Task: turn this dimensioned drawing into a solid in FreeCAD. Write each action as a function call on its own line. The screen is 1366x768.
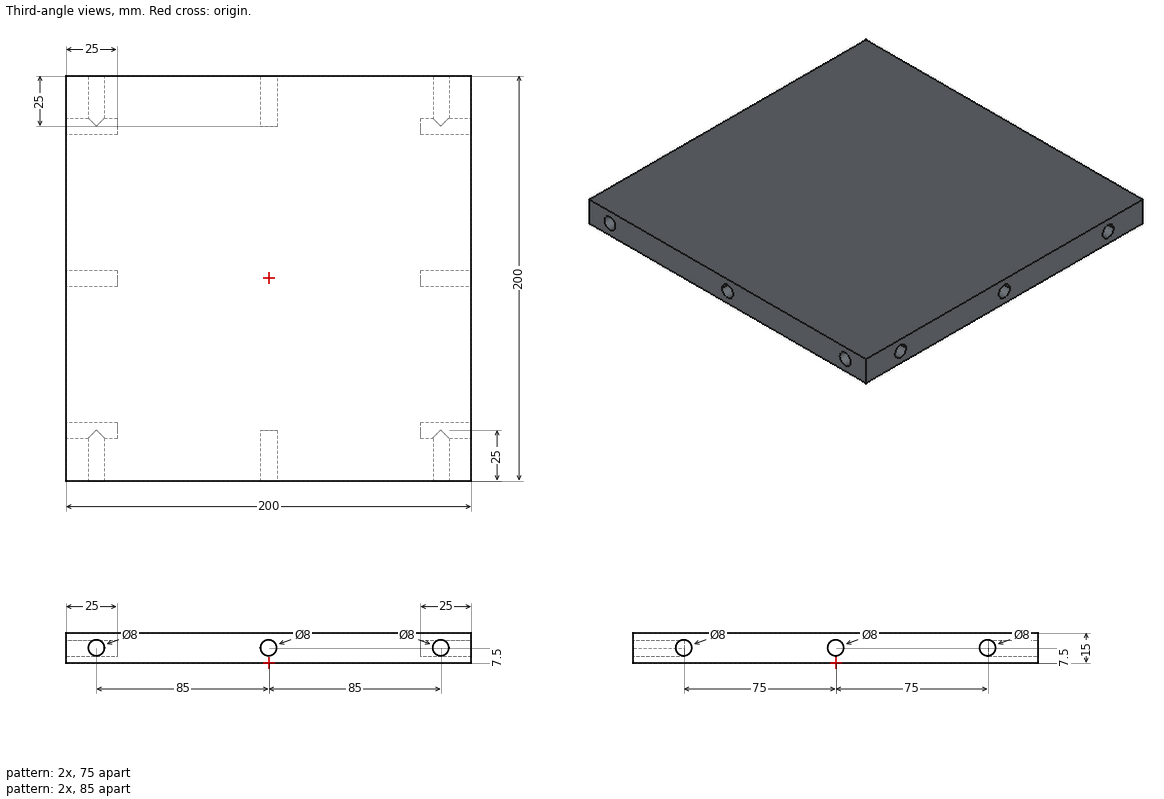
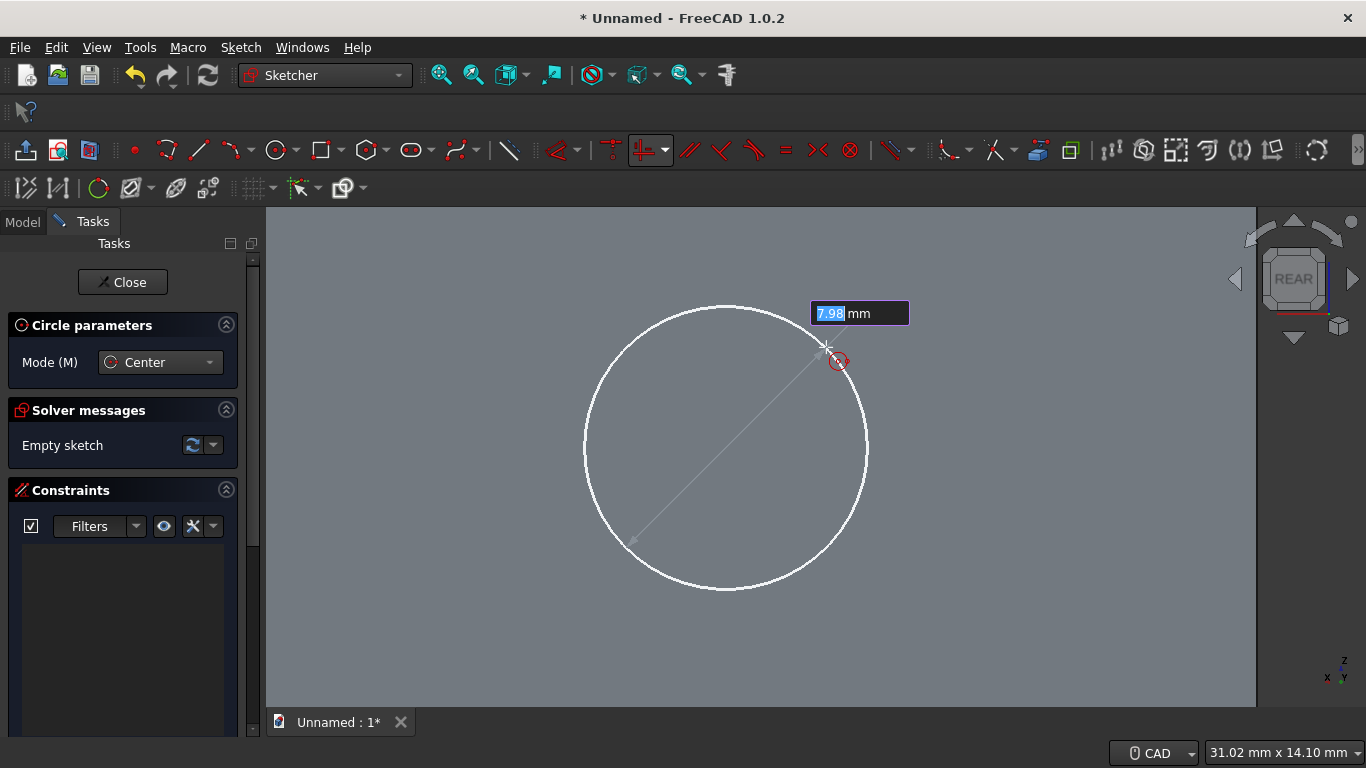
text(8)
key(Return)
key(Escape)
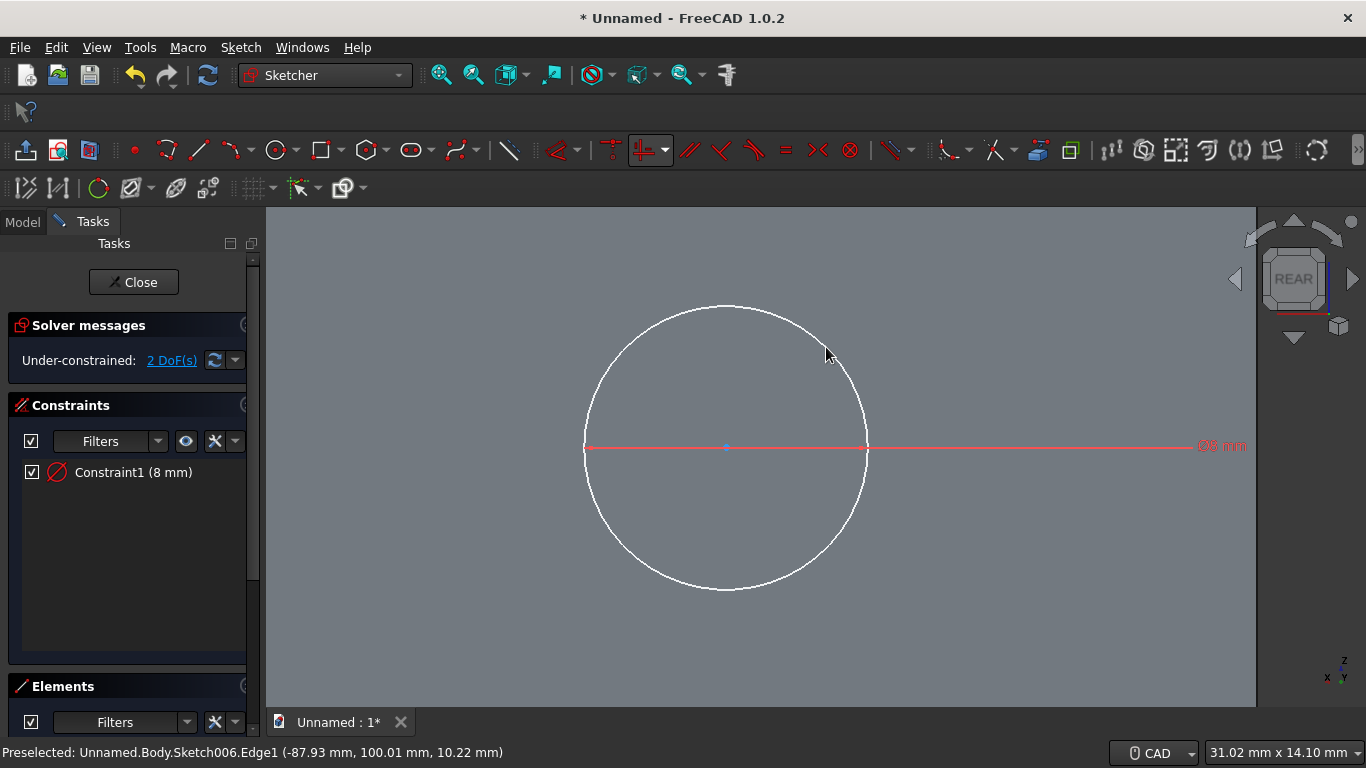
key(d)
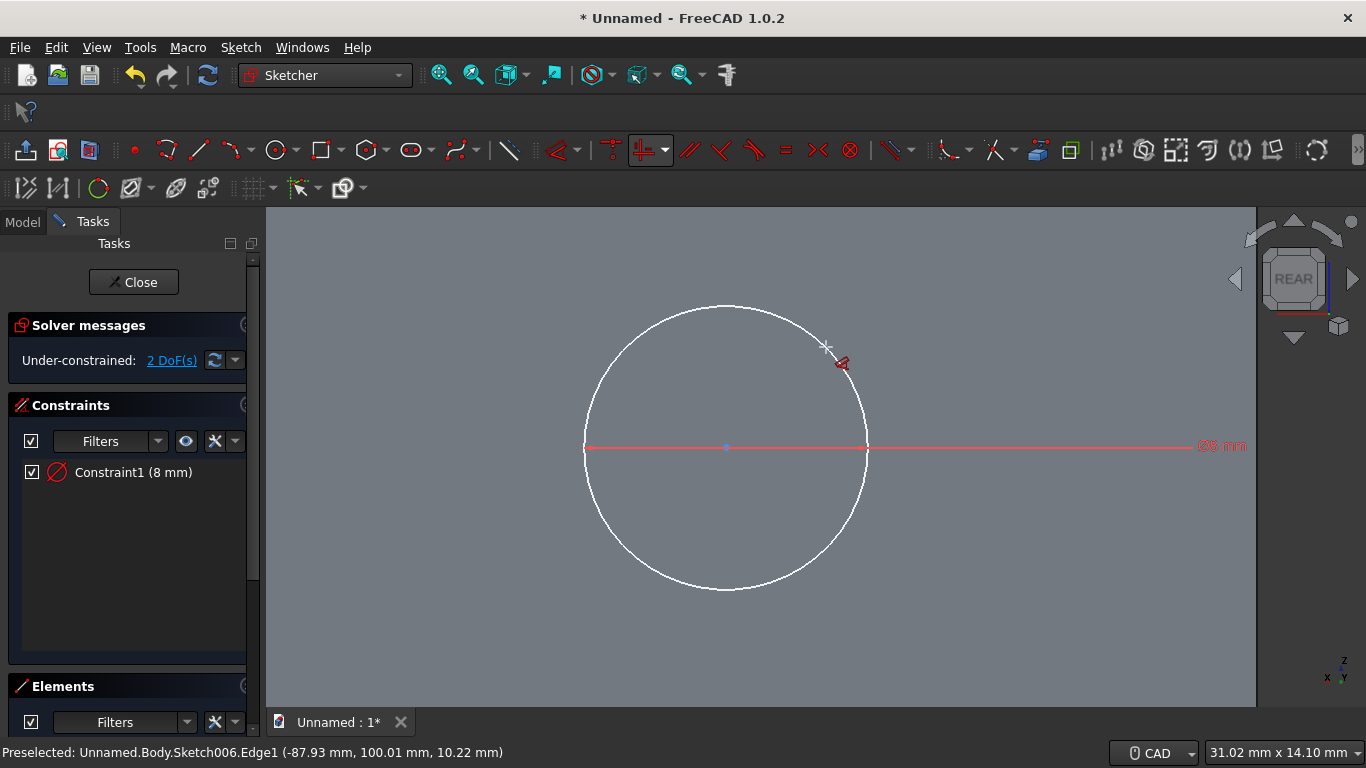
click(726, 448)
click(510, 414)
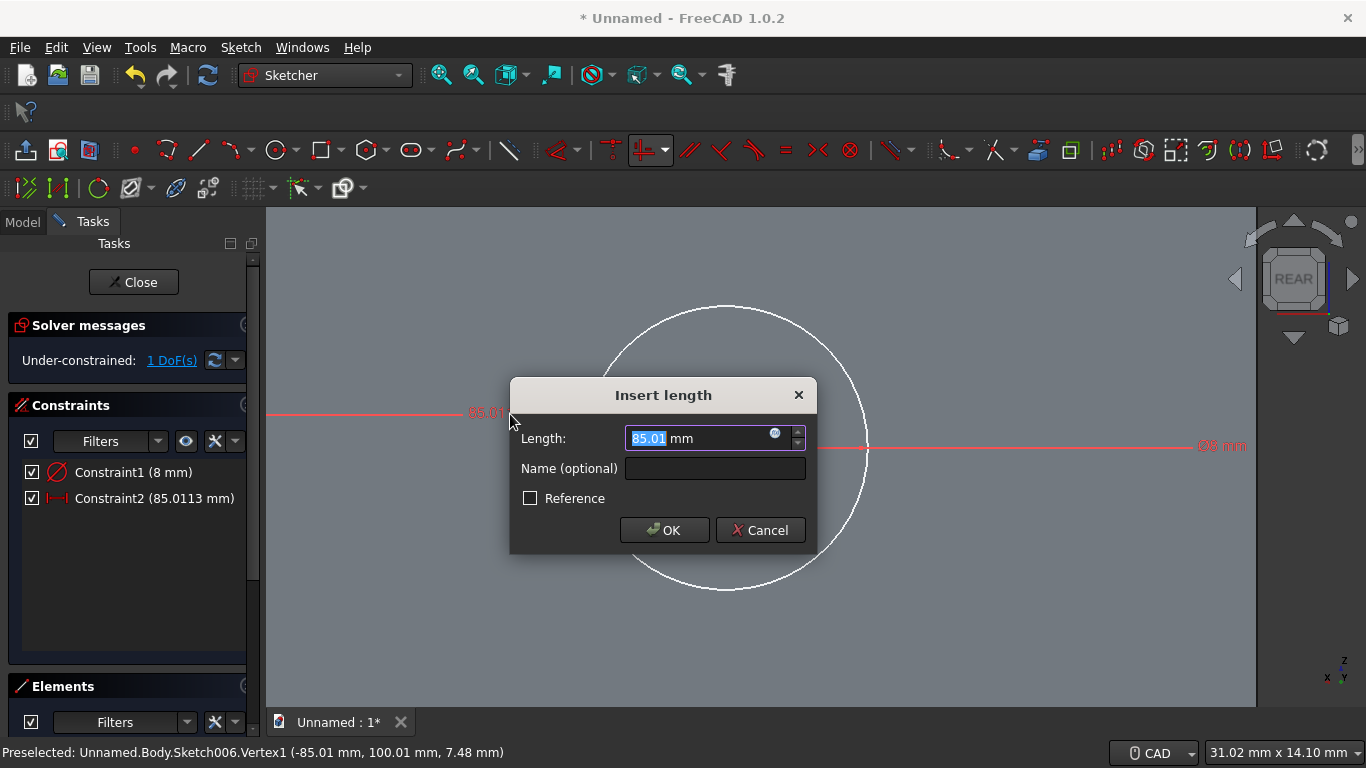
text(85)
key(Return)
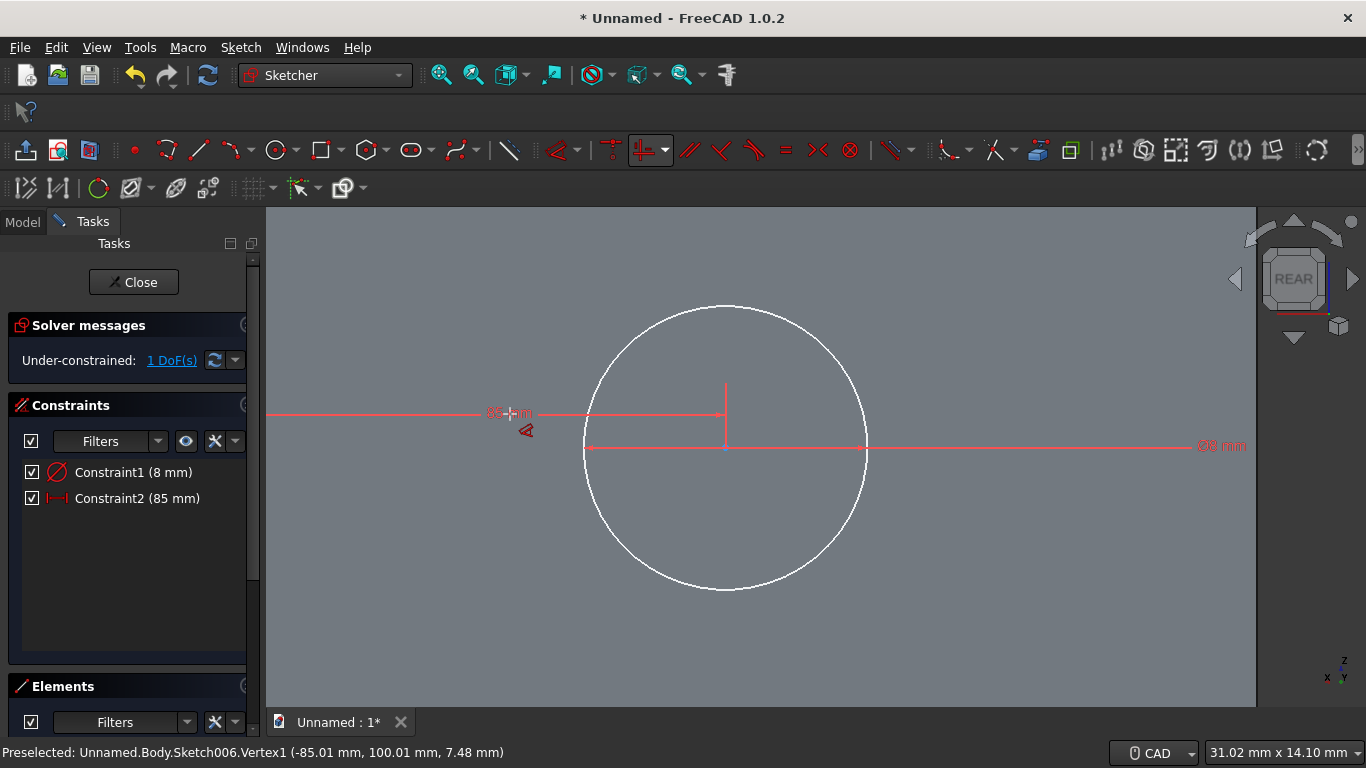
click(726, 448)
click(760, 563)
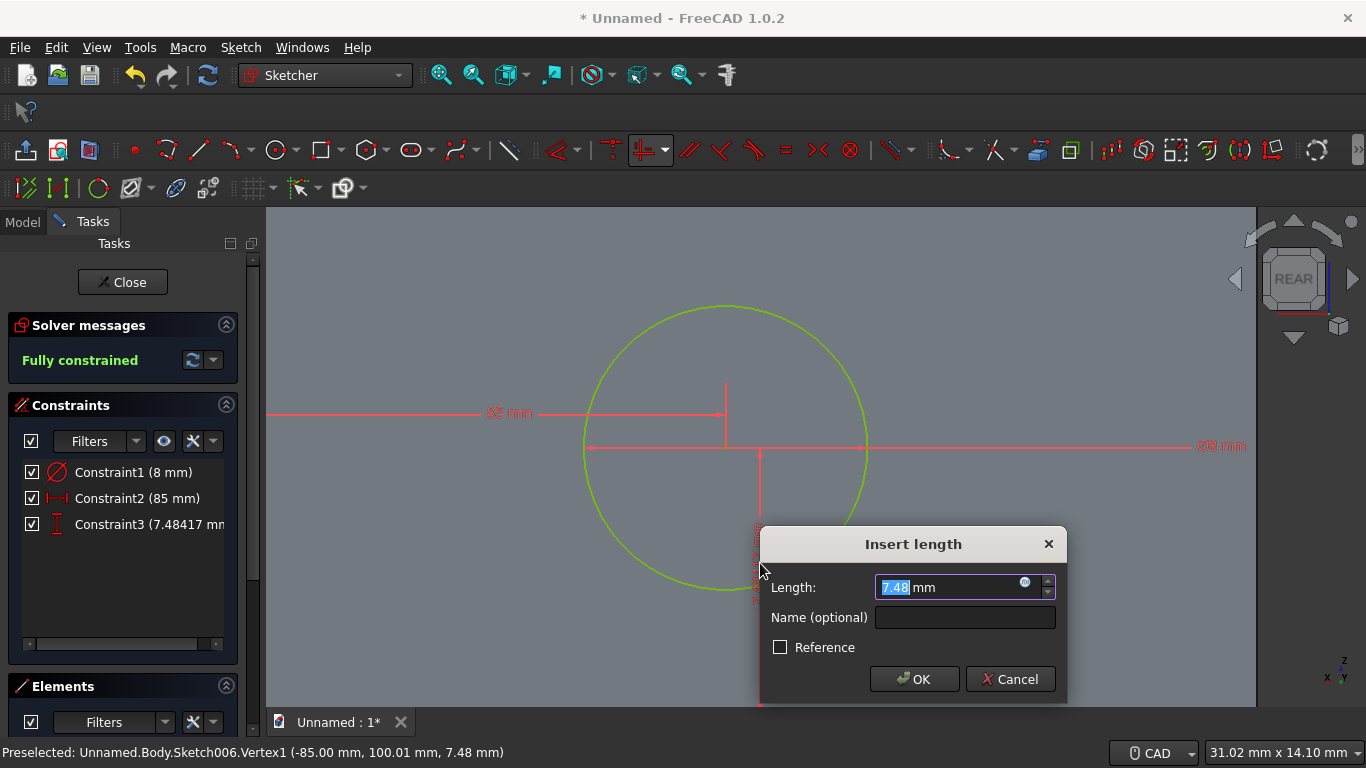
text(7.5)
key(Return)
key(Escape)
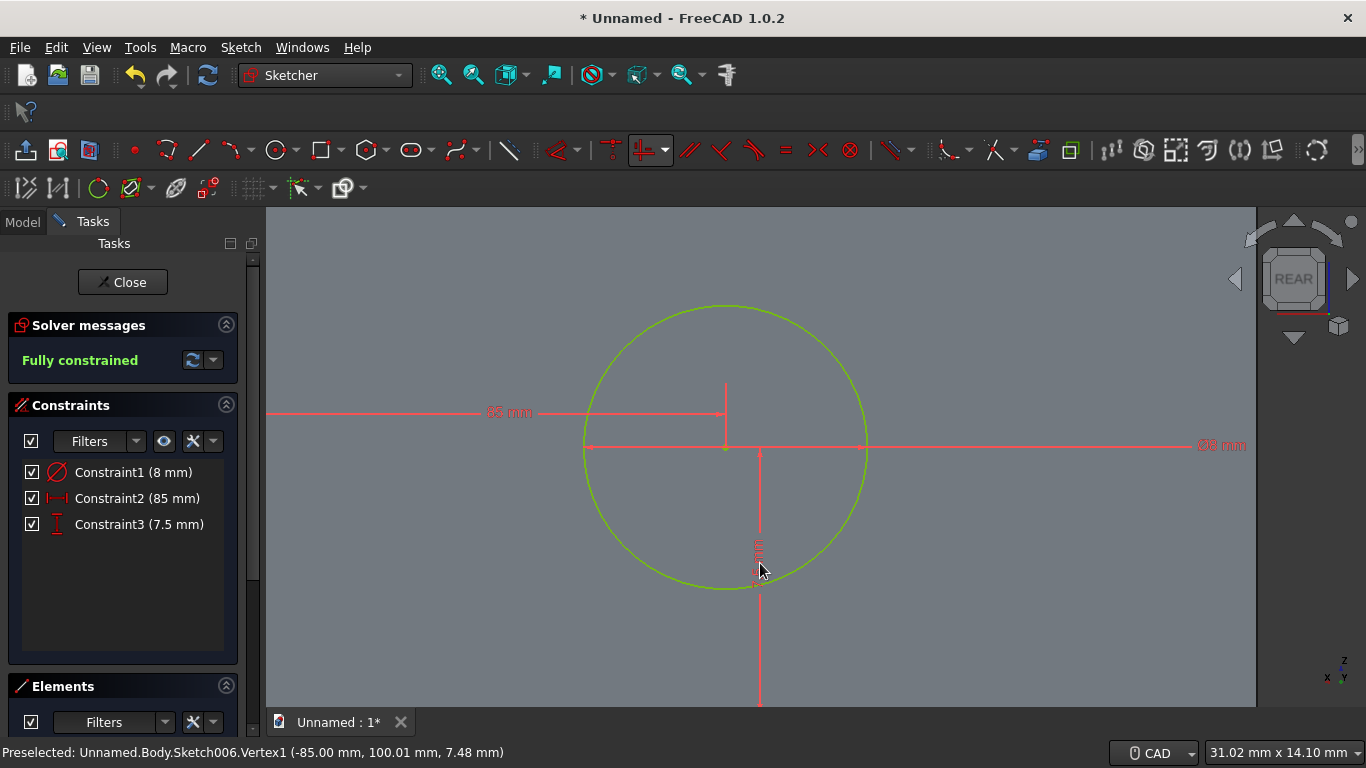
click(123, 282)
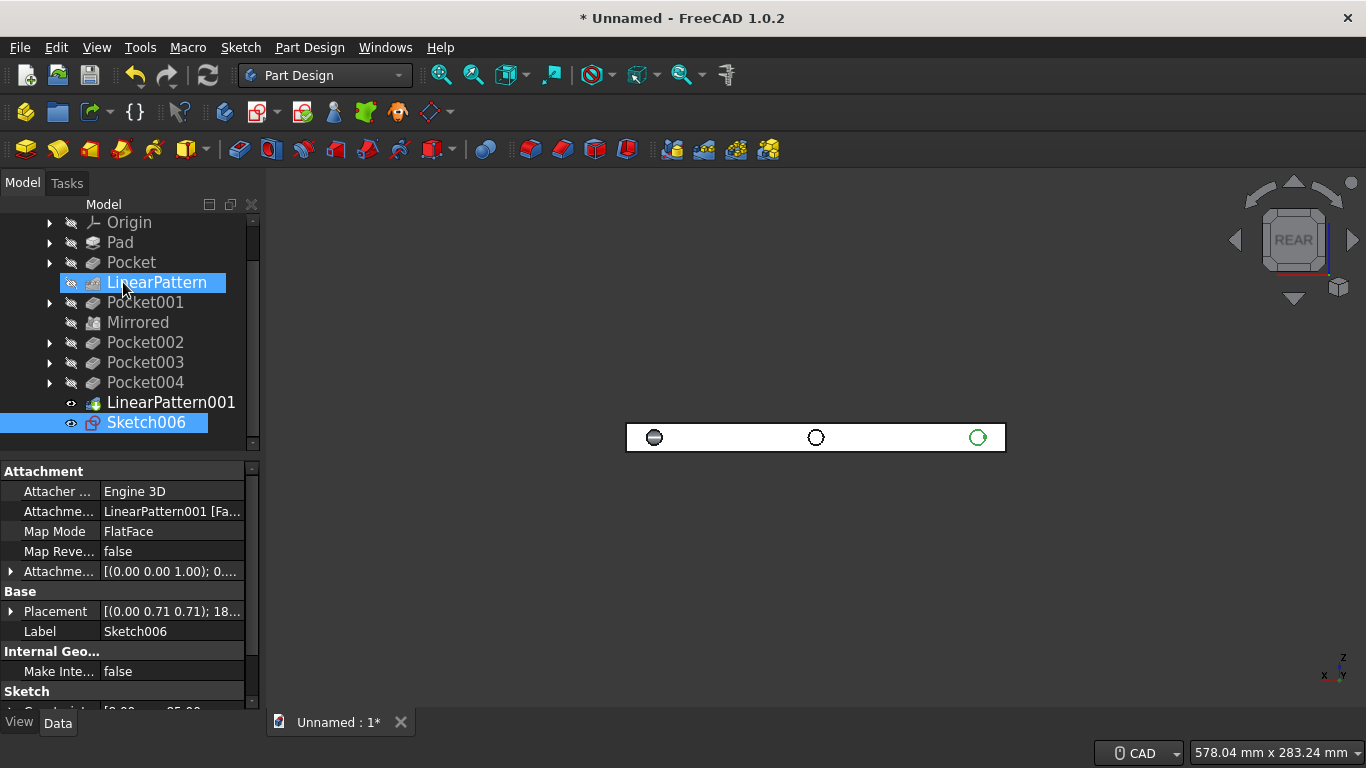
click(240, 150)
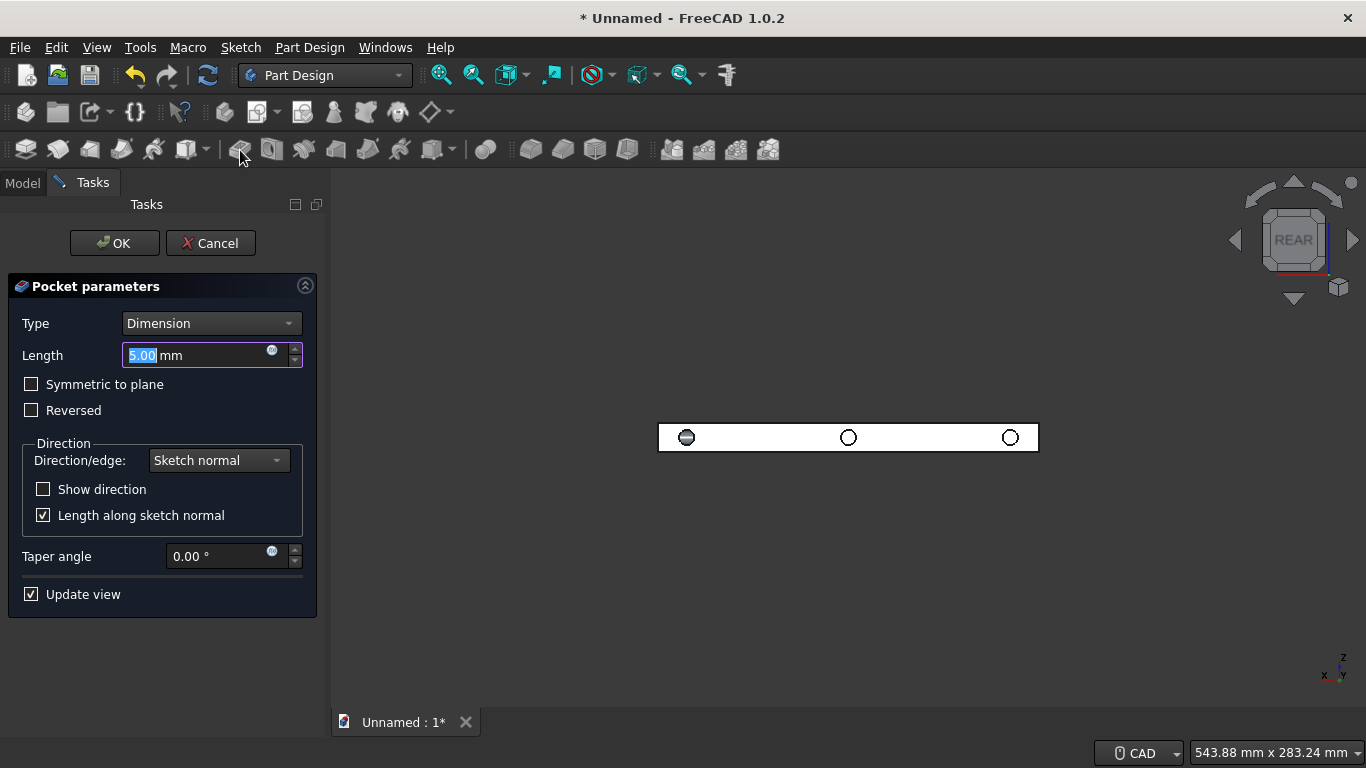
text(25)
key(Tab)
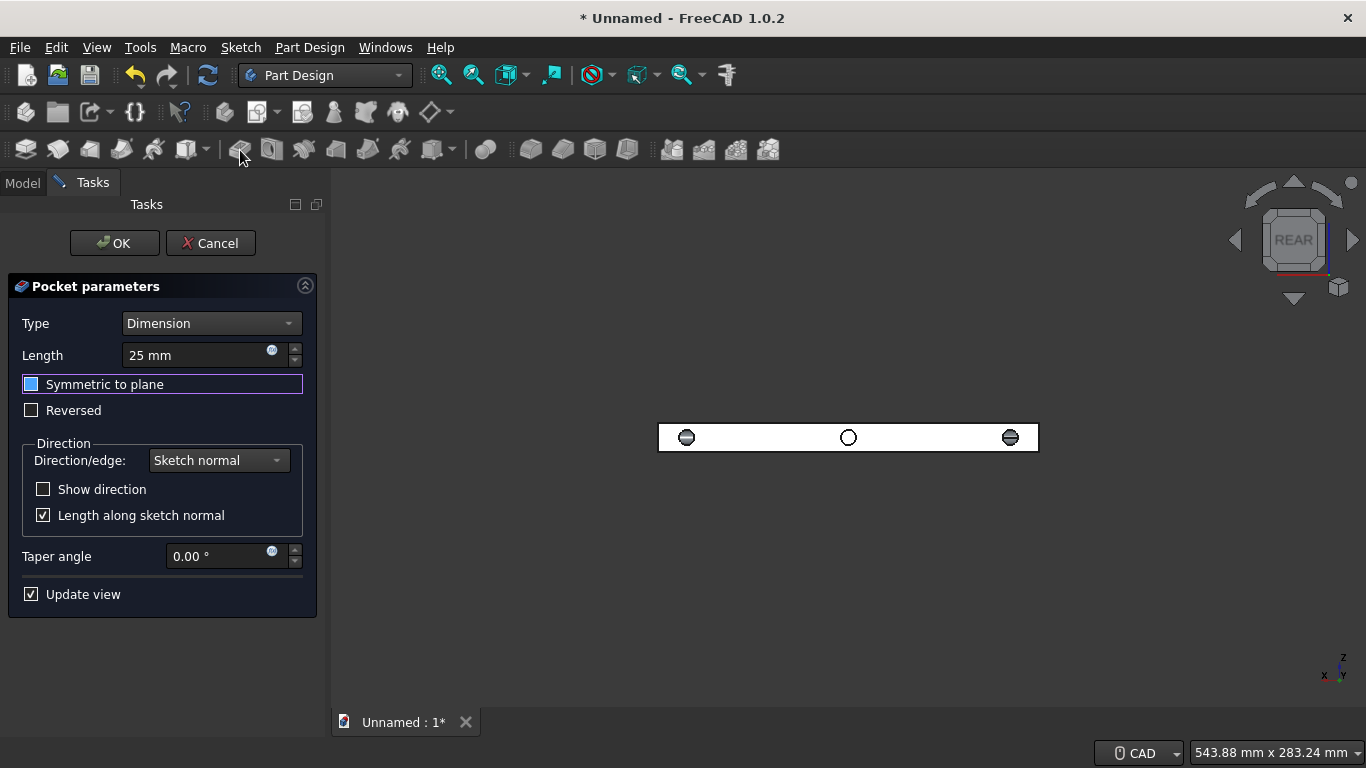
click(115, 243)